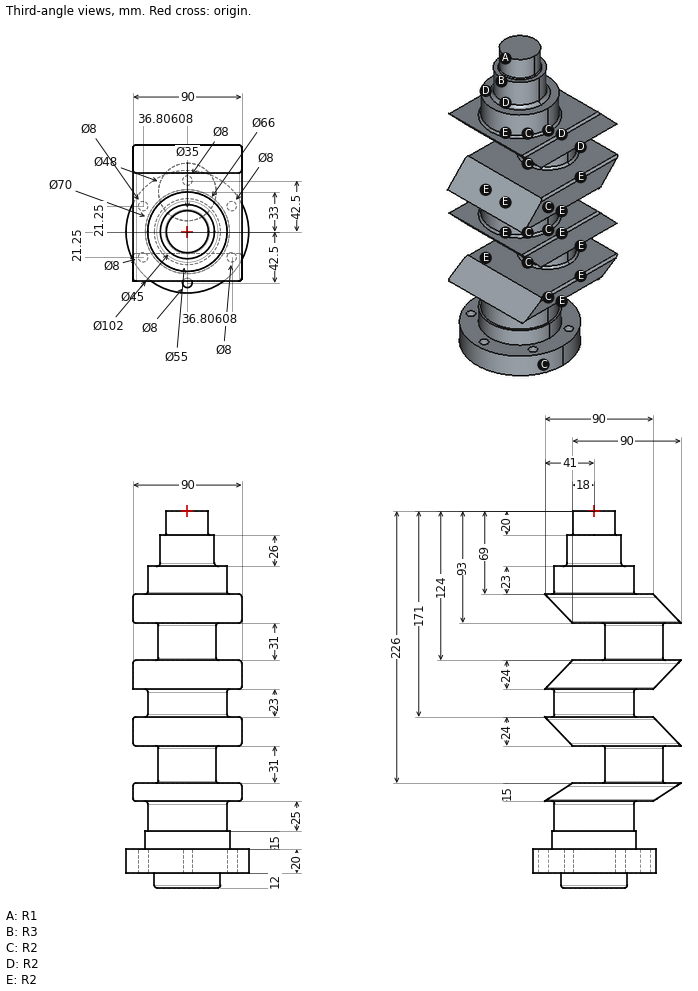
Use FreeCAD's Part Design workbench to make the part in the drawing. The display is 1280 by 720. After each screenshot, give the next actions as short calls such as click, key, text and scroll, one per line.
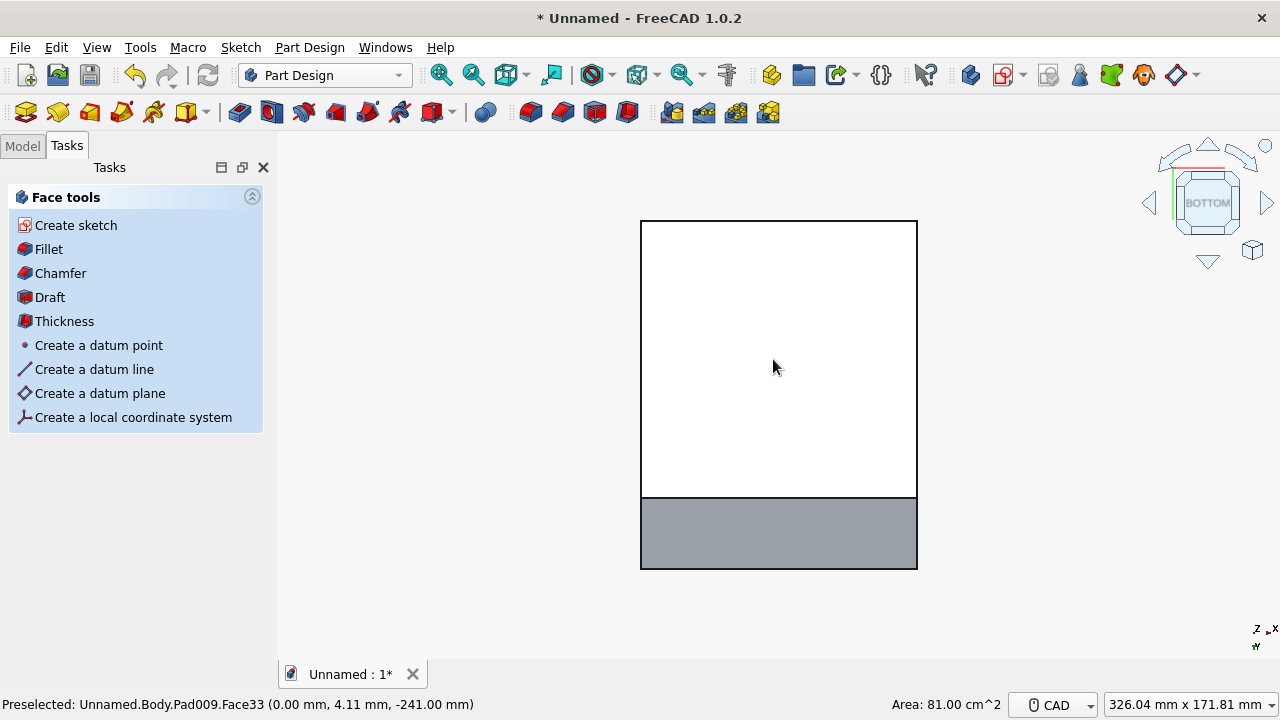
click(1004, 76)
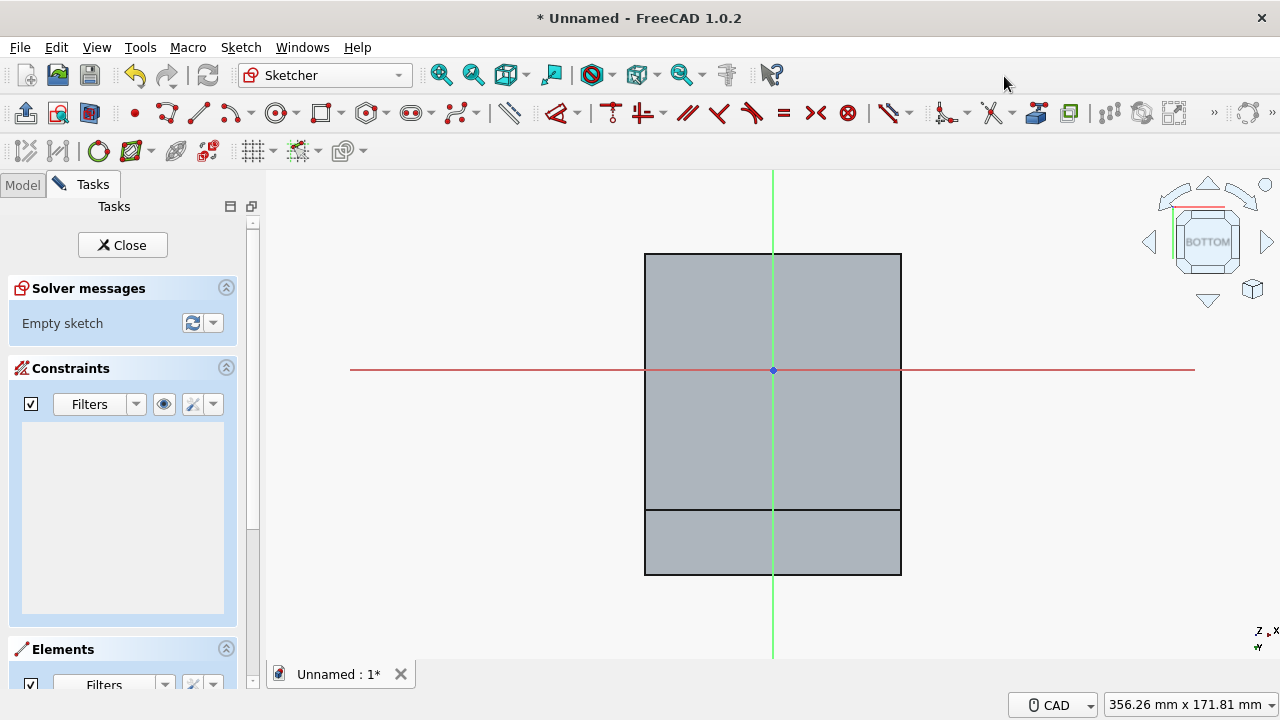
scroll(912, 281, up, 2)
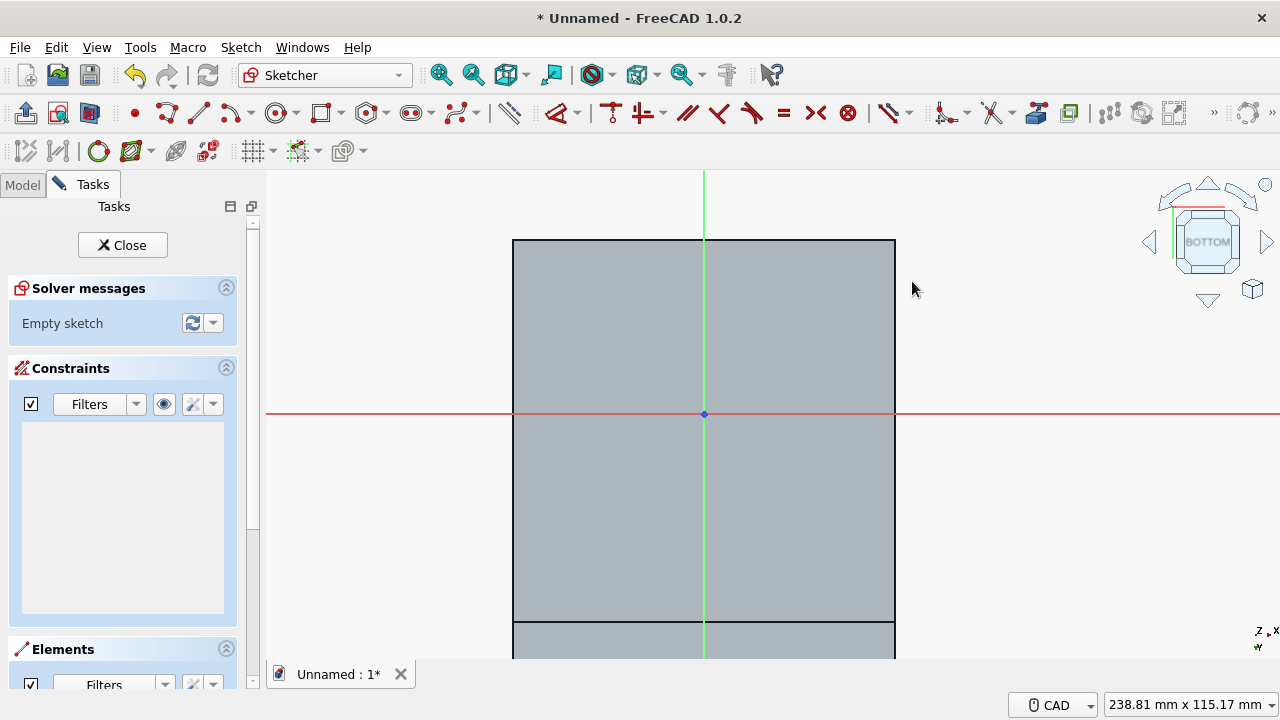
click(276, 114)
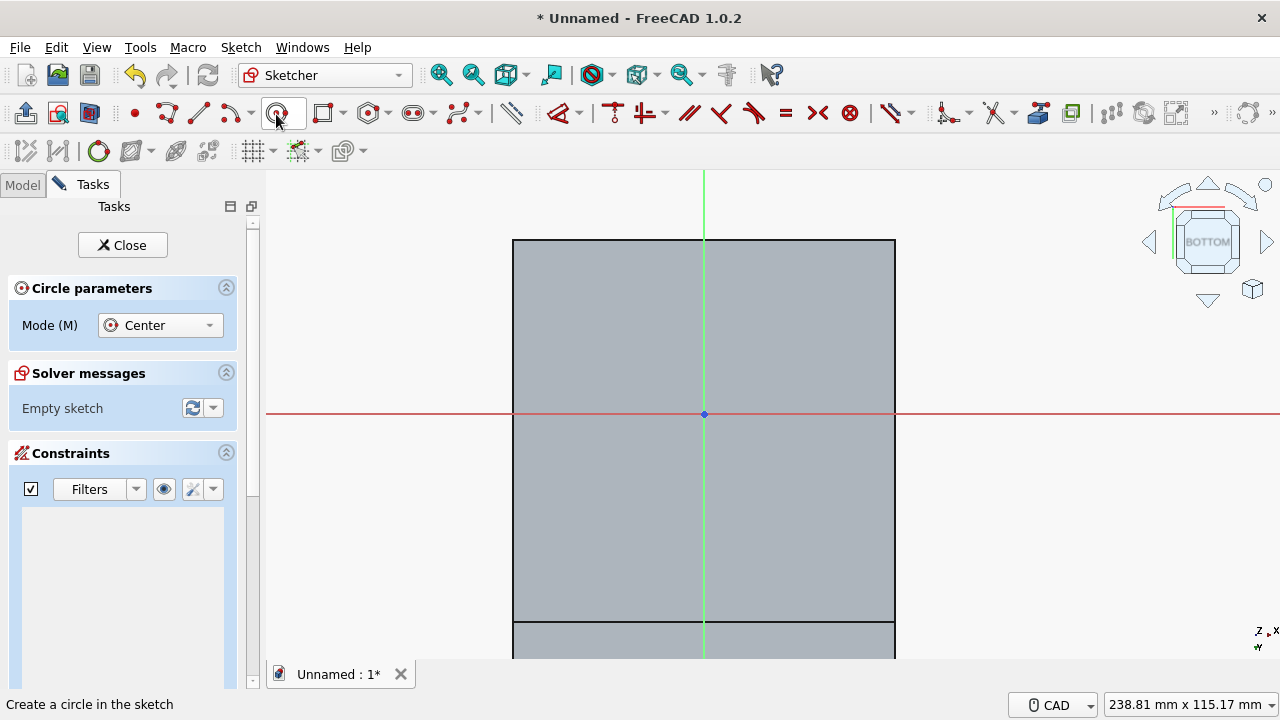
click(704, 414)
move(803, 315)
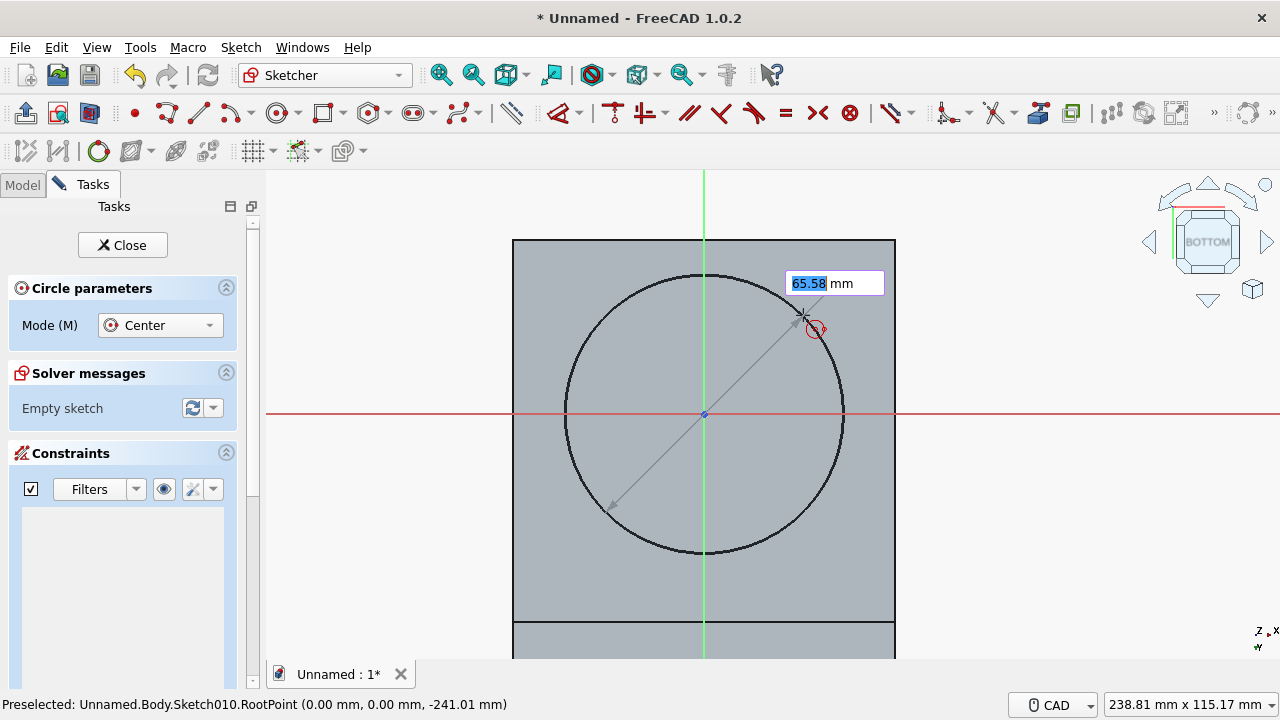
text(66)
key(Return)
key(Escape)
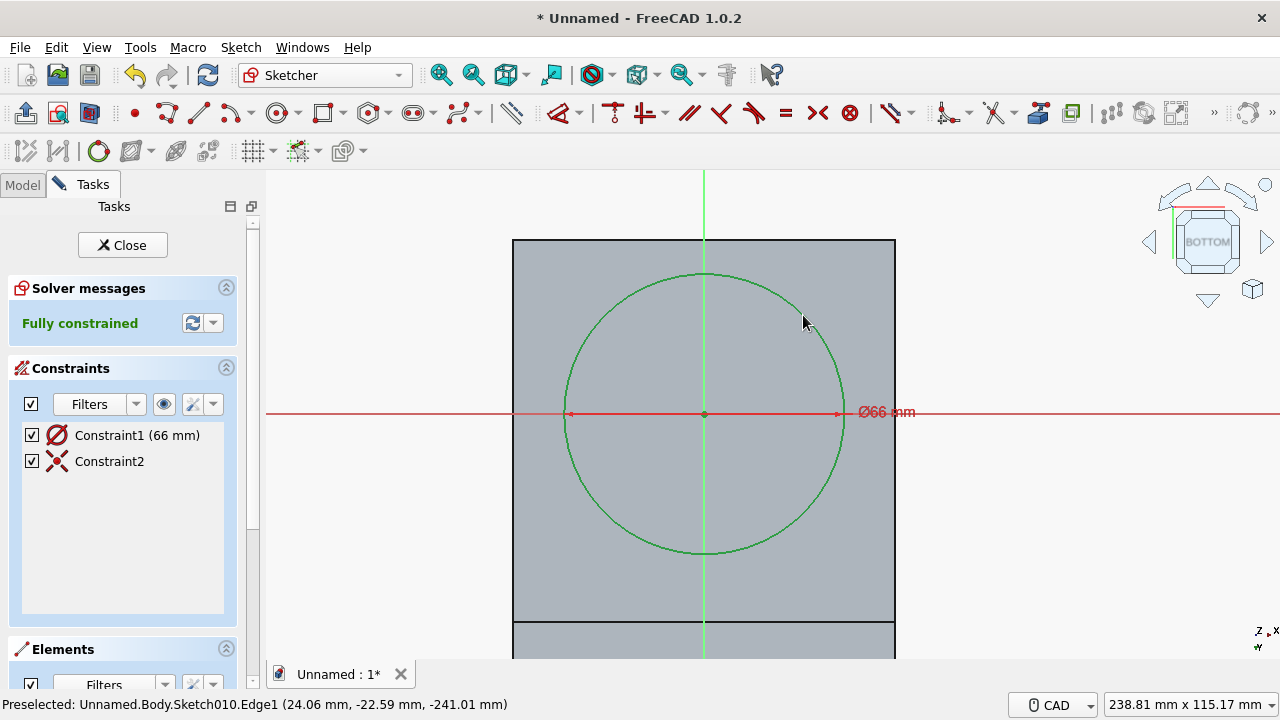
click(123, 245)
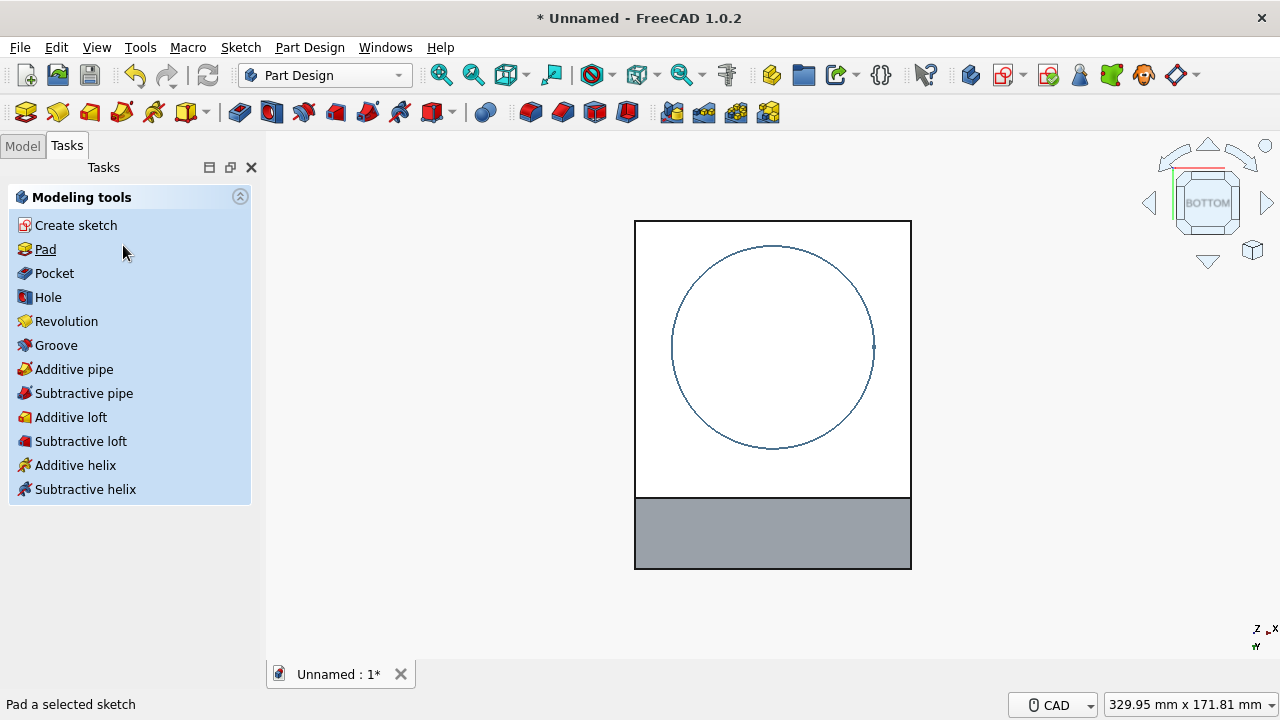
click(26, 112)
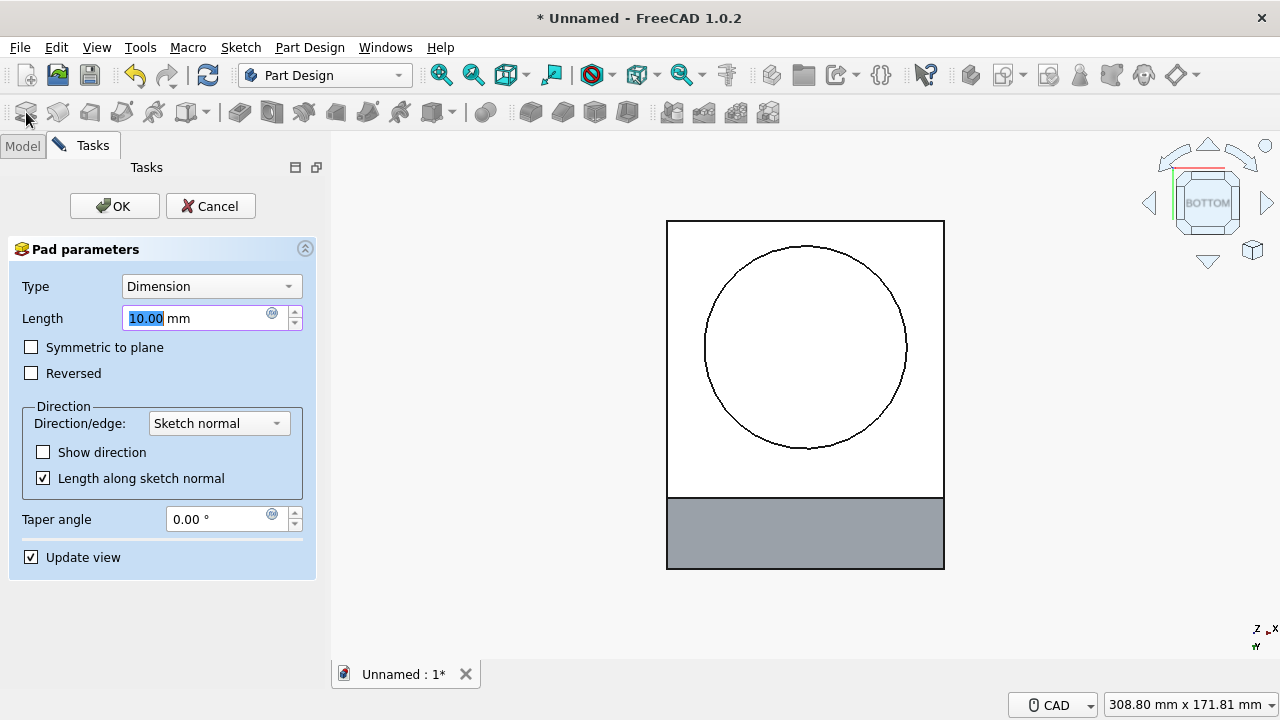
text(25)
key(Tab)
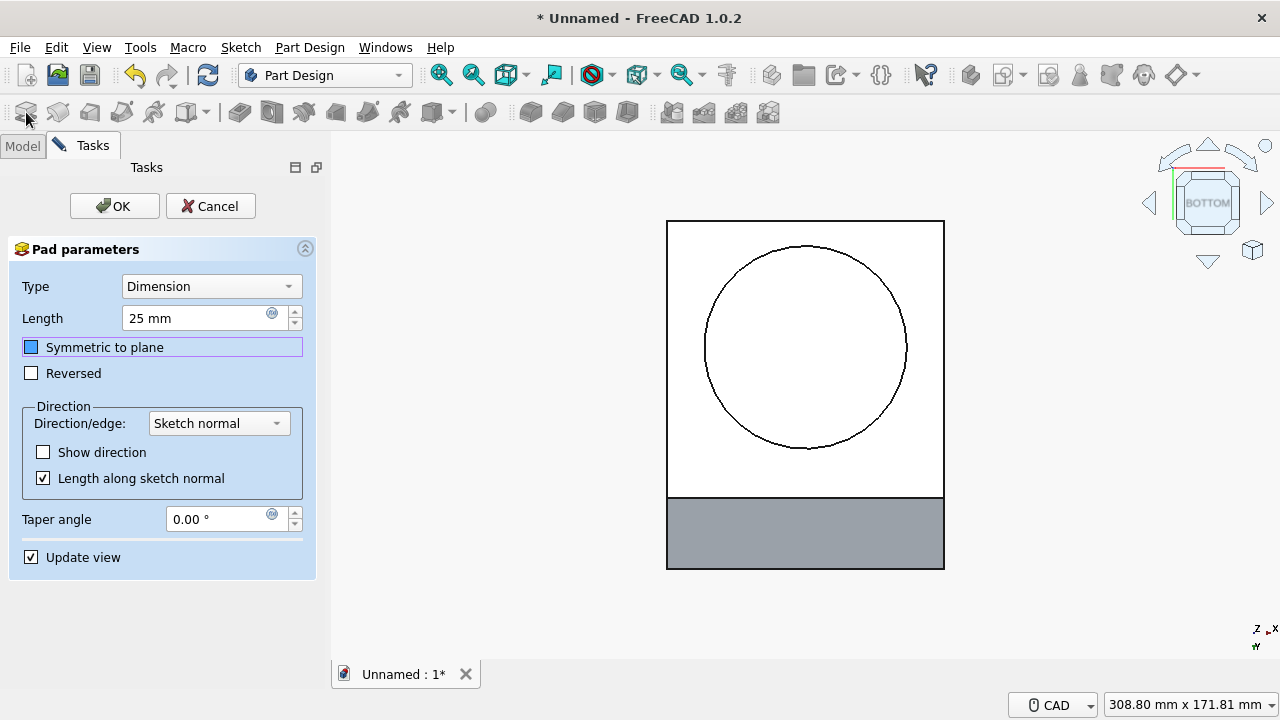
click(115, 206)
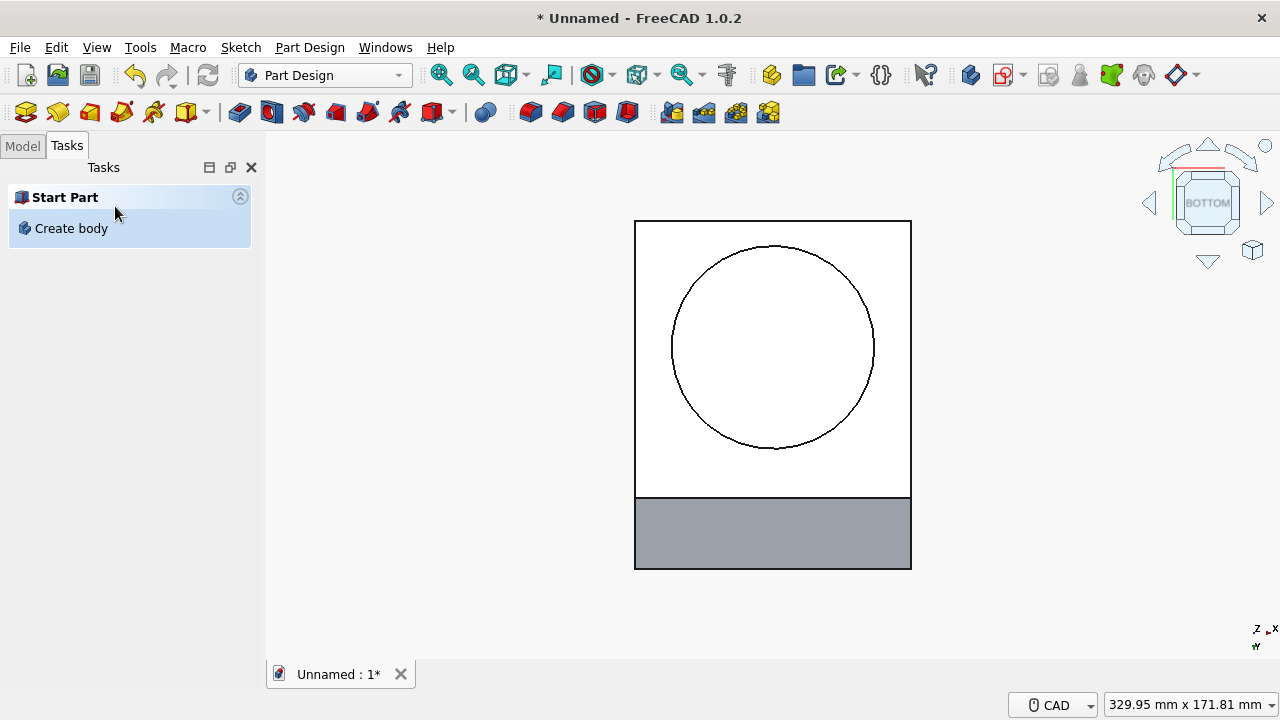
click(773, 346)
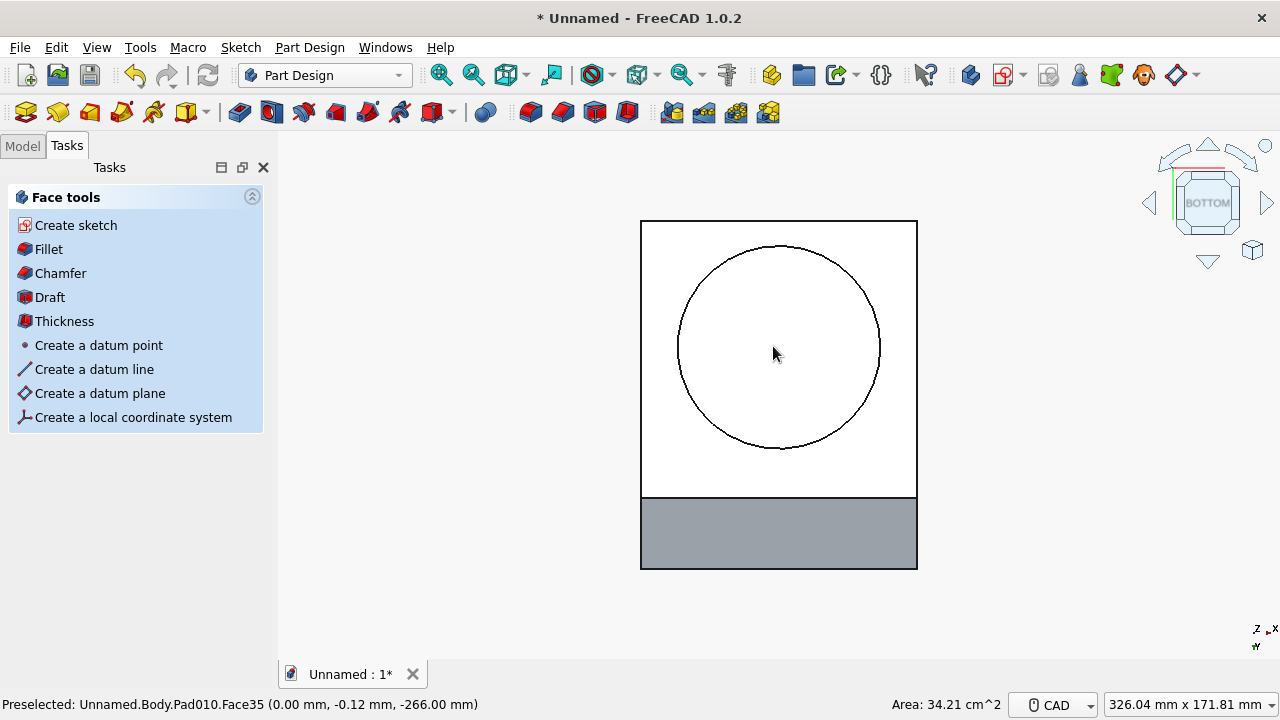
click(1004, 76)